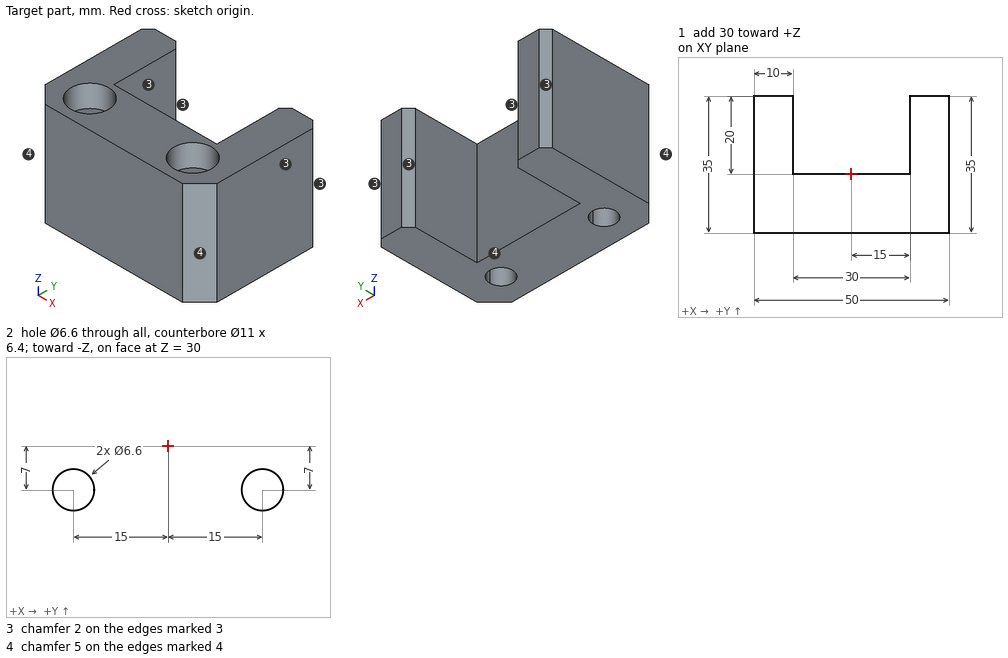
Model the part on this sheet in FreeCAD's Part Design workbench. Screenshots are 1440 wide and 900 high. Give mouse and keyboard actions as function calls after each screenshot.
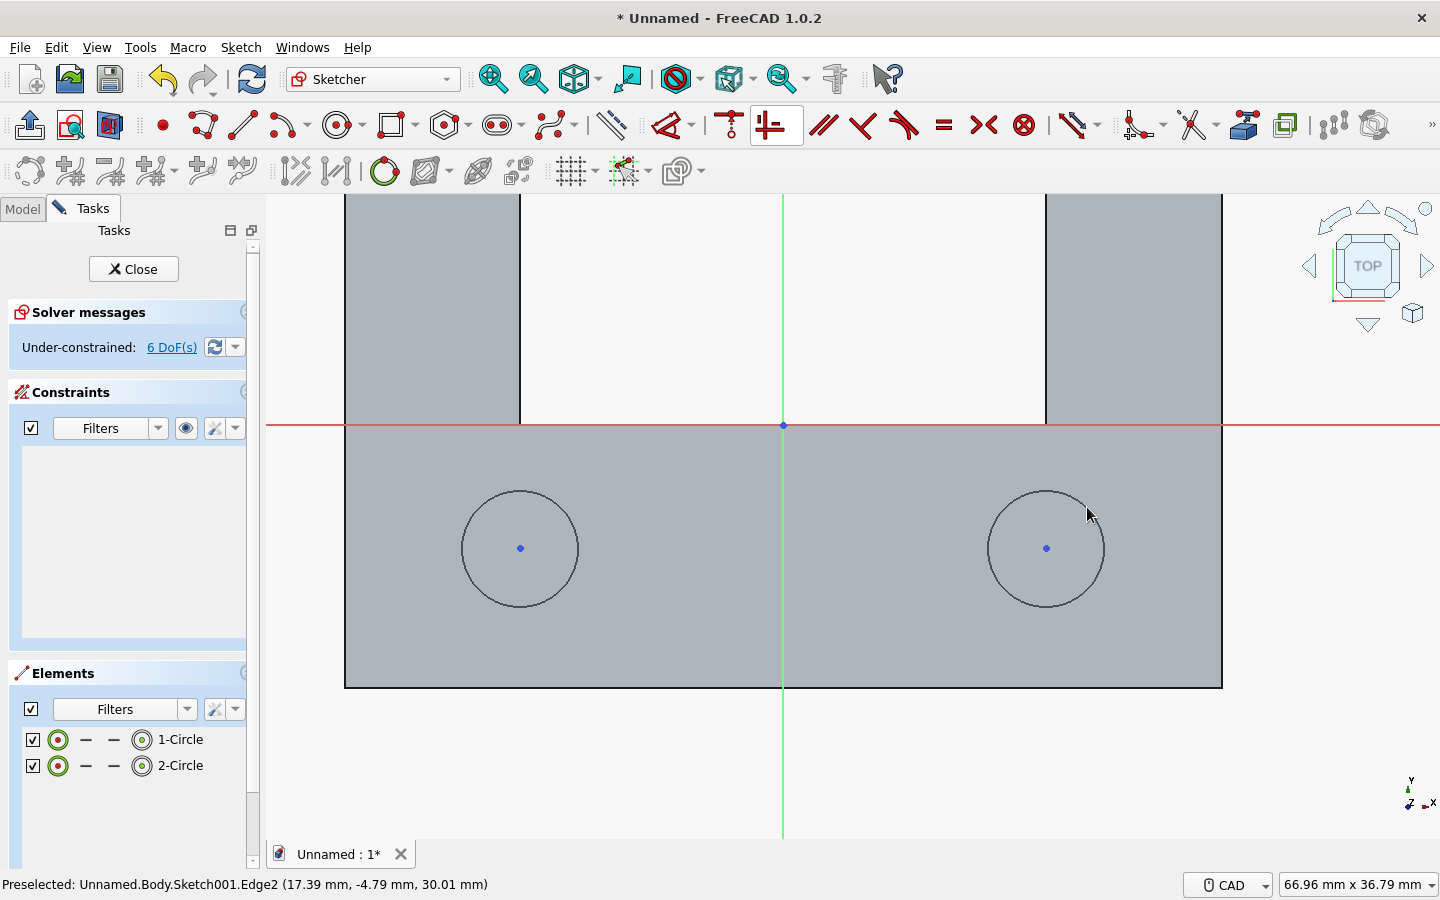
click(561, 508)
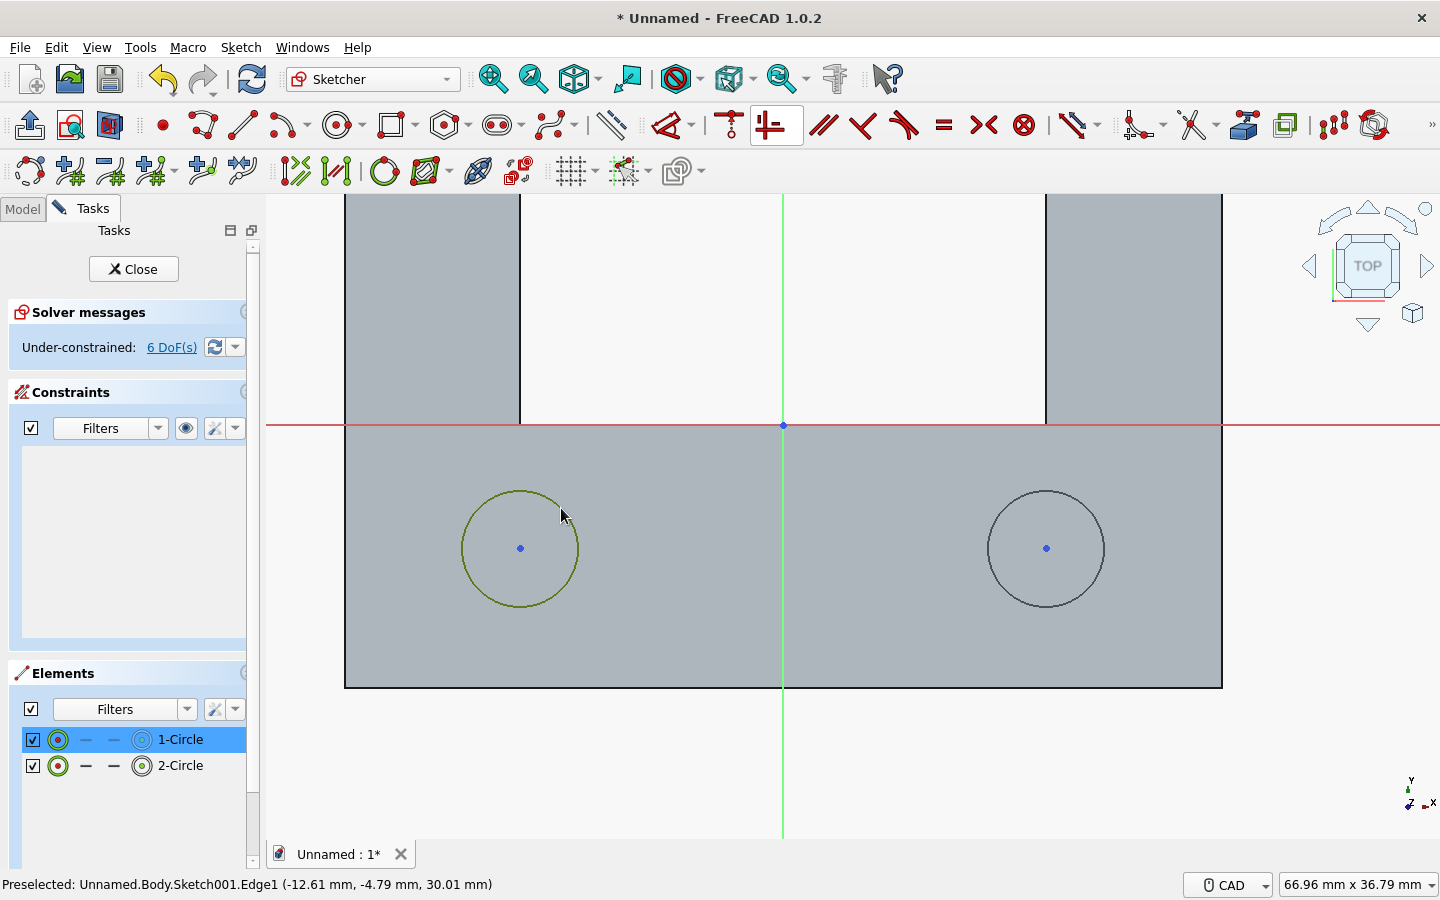
click(1087, 508)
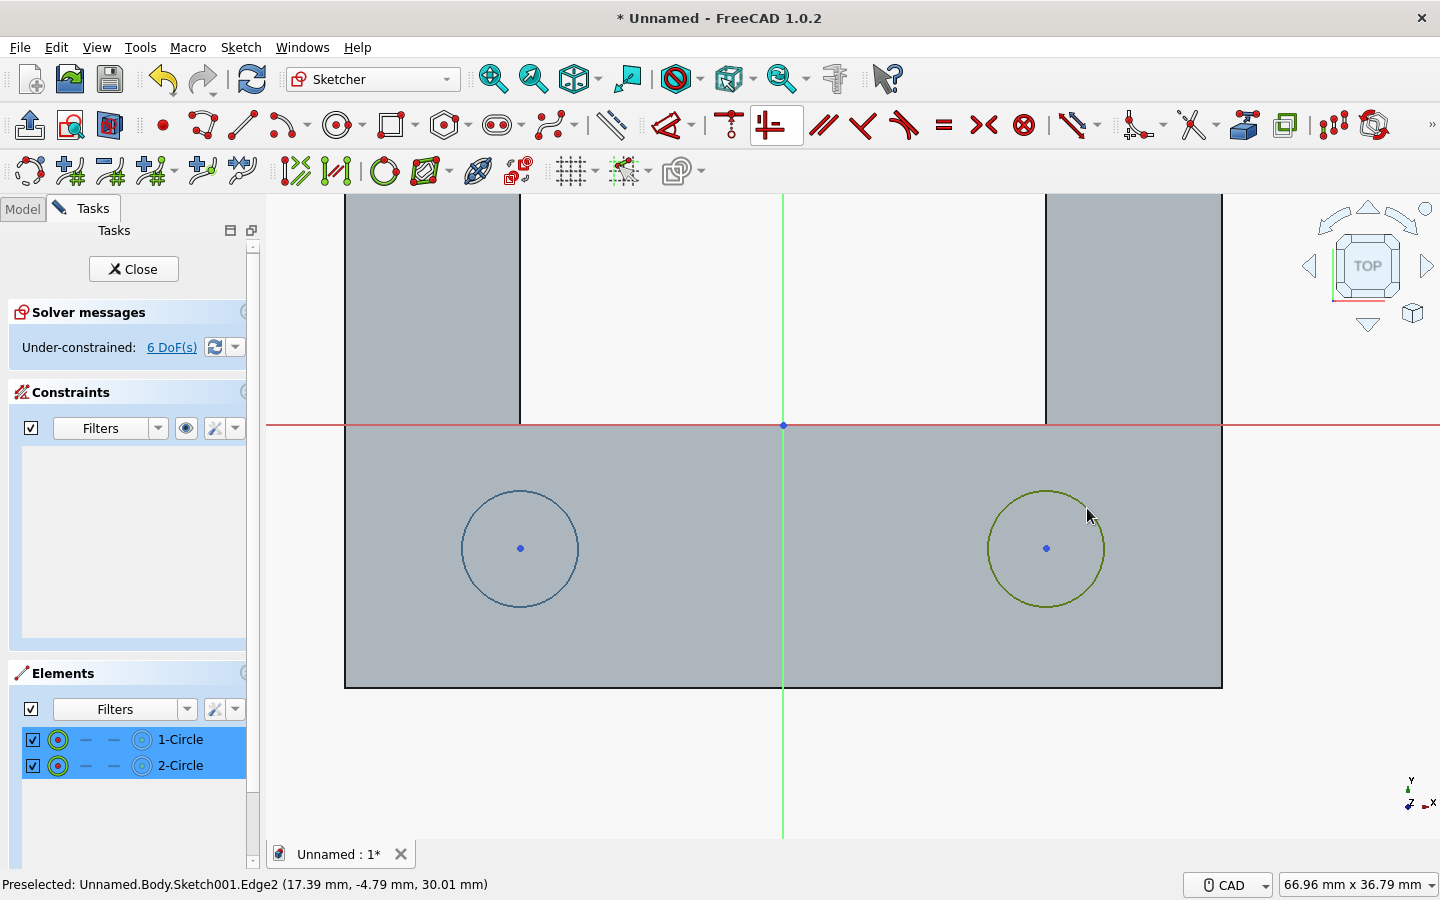
click(944, 126)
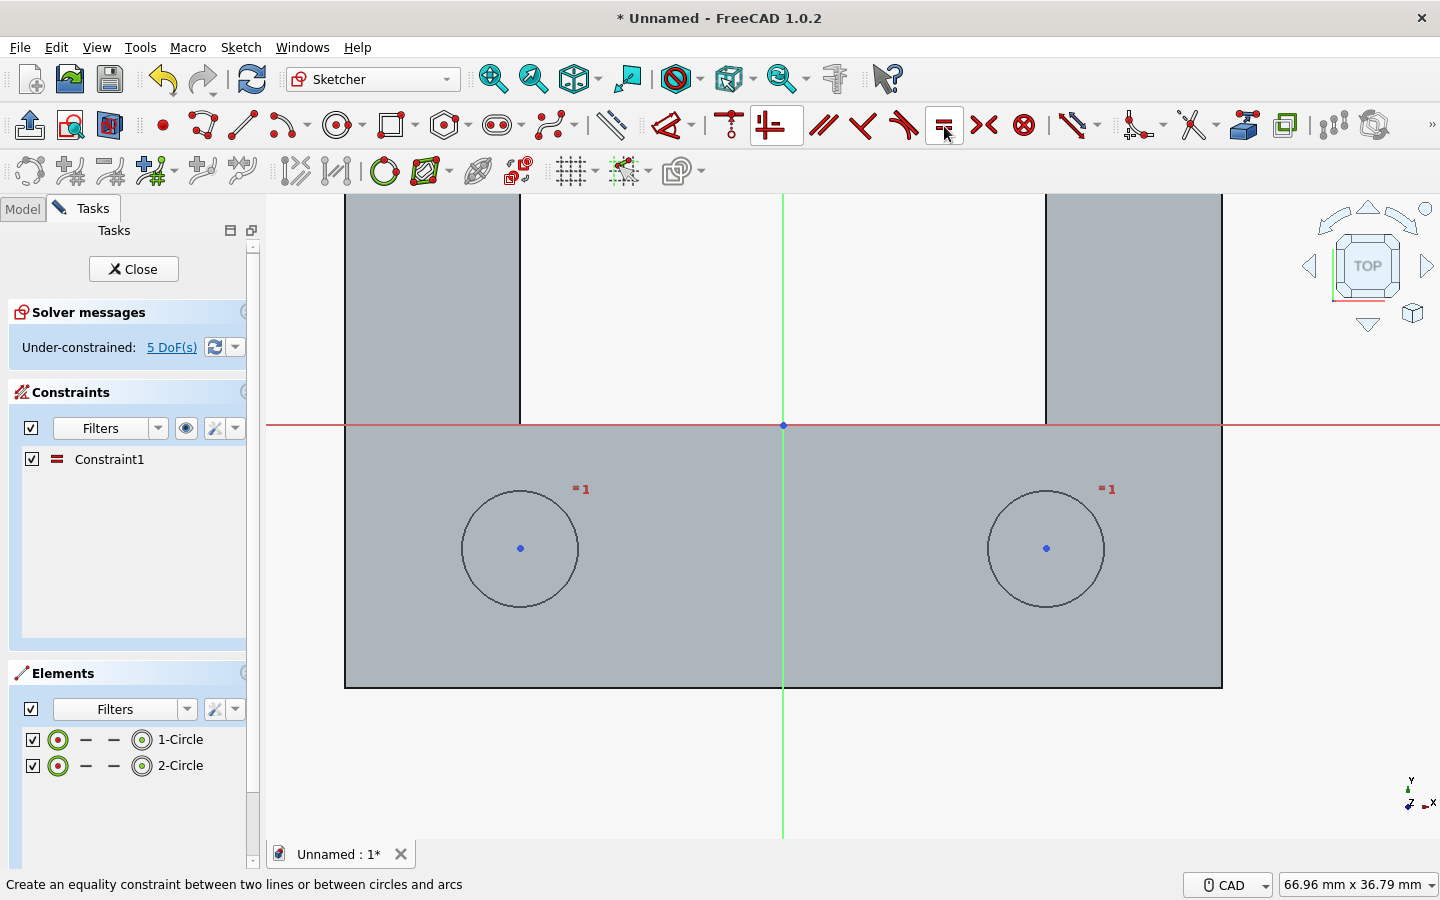
click(666, 126)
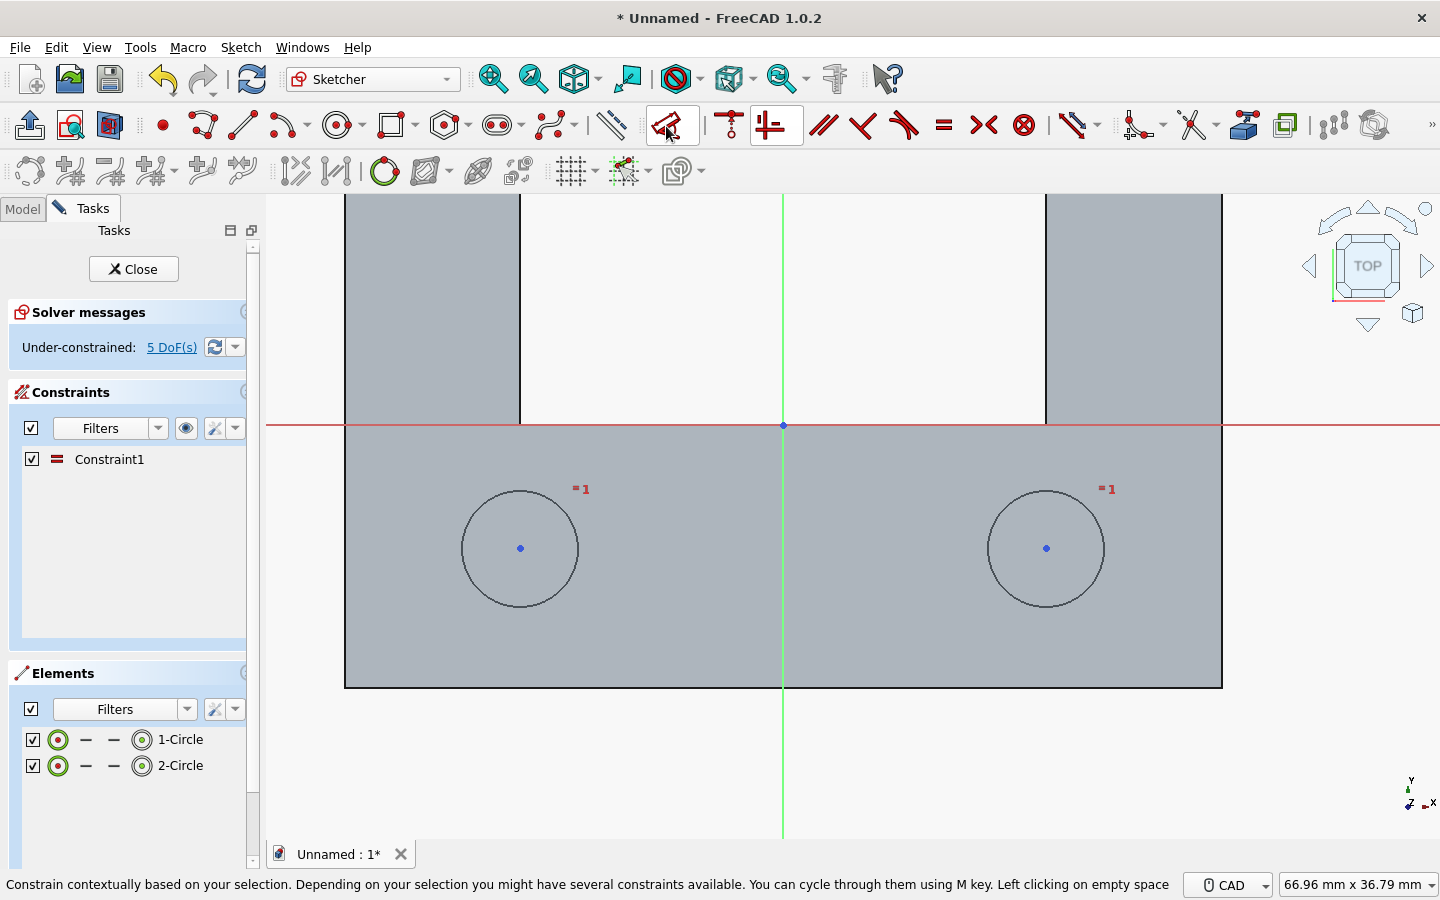
click(561, 508)
click(584, 485)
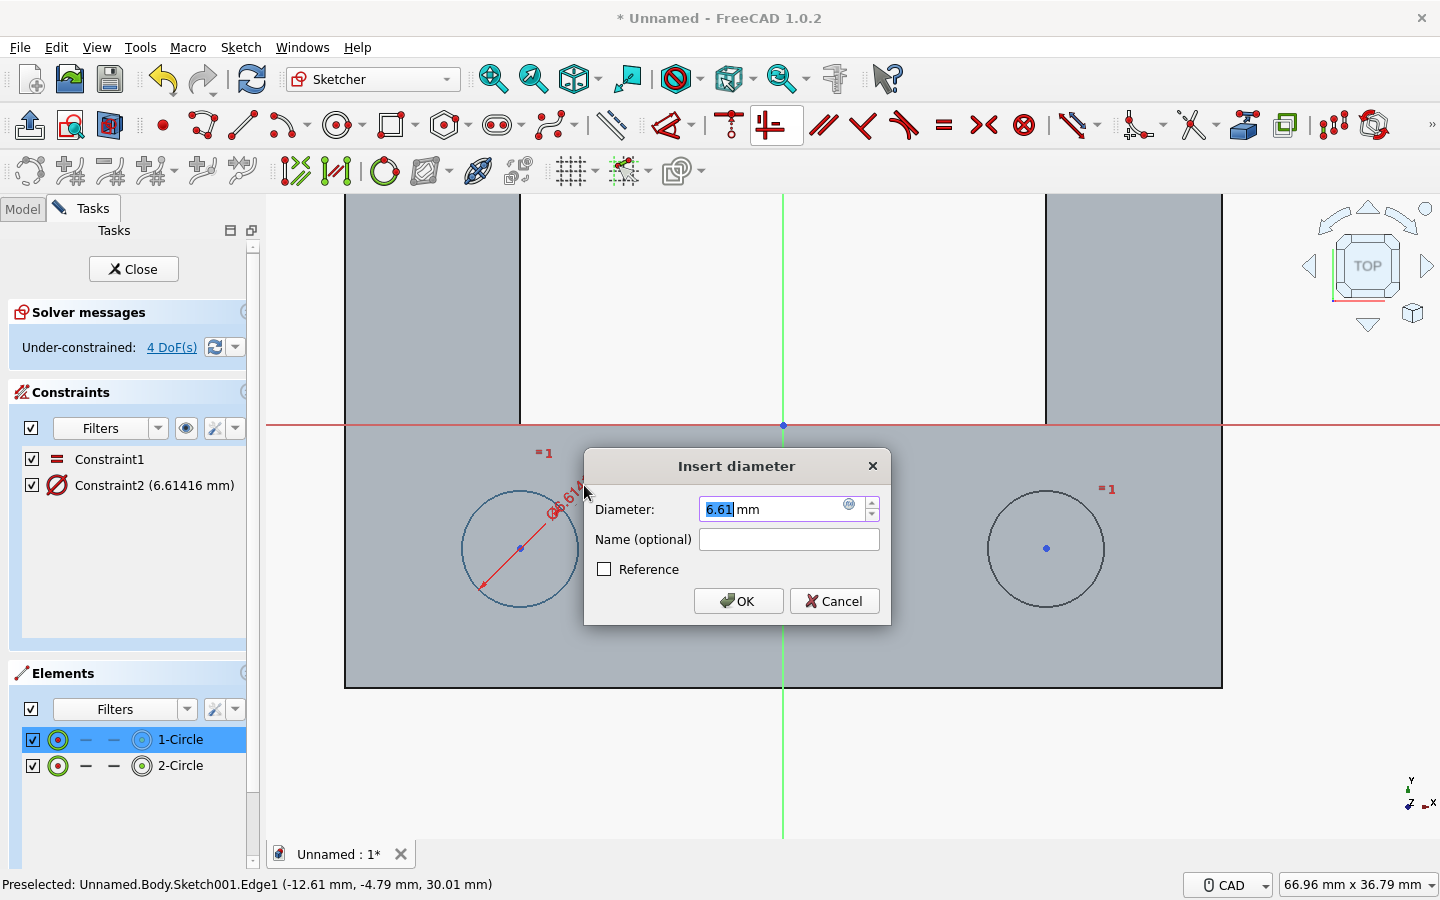
text(6.6)
key(Return)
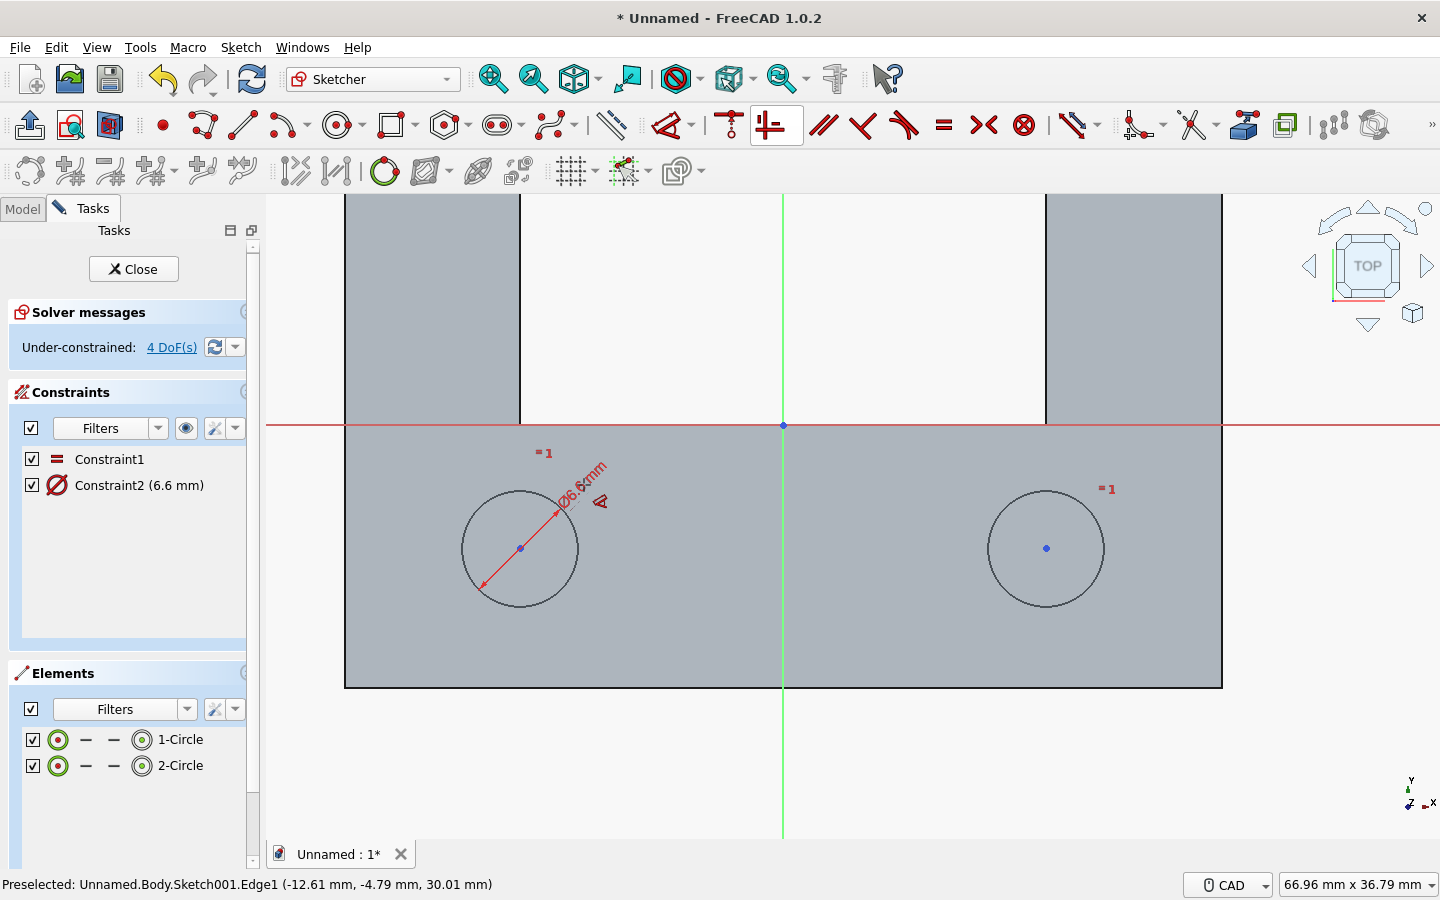
click(520, 549)
click(486, 459)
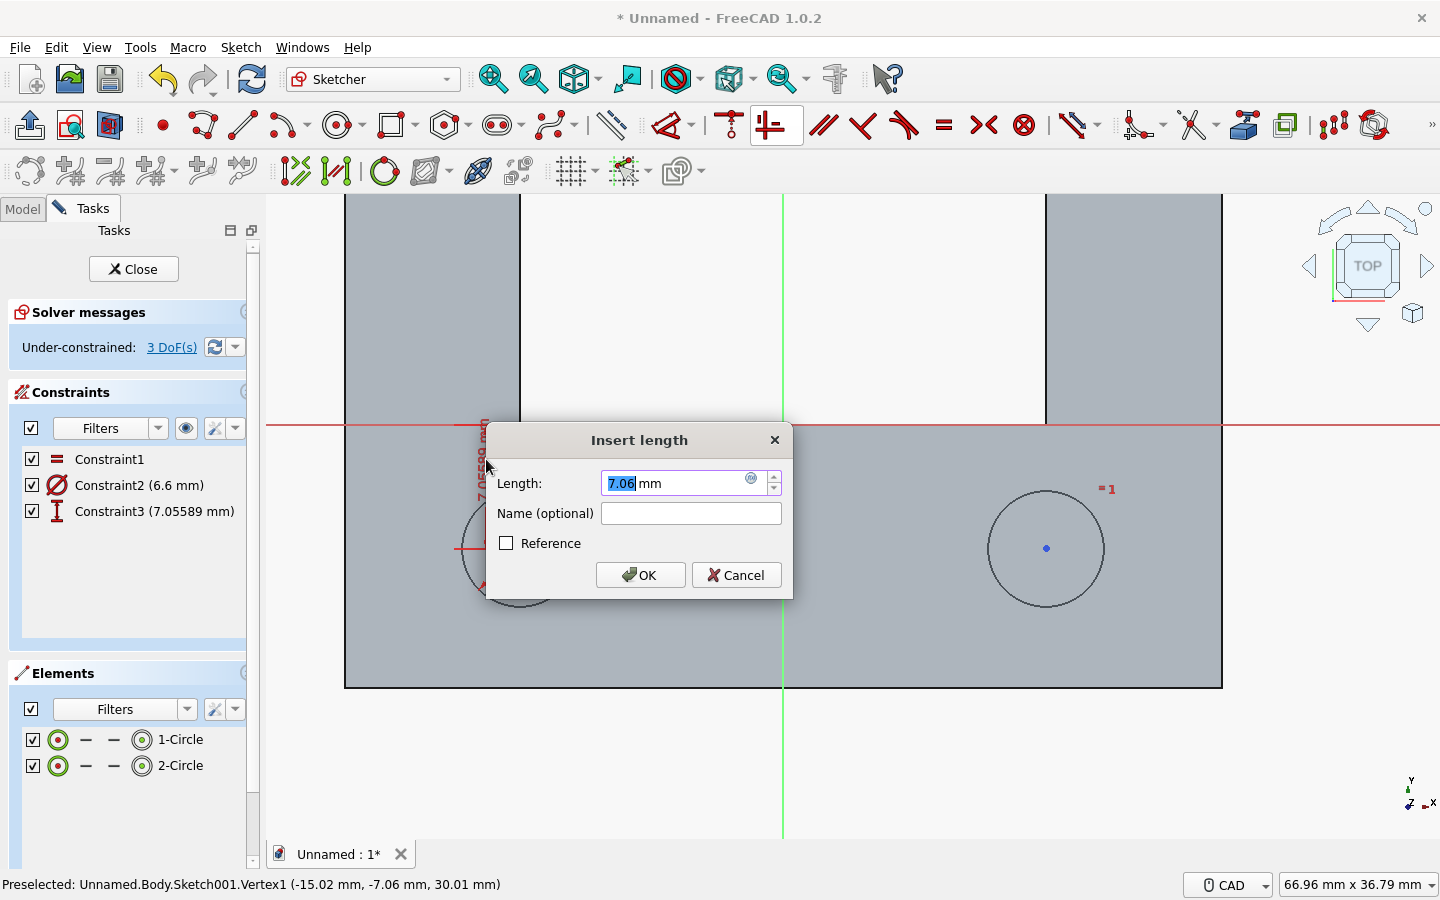
text(7)
key(Return)